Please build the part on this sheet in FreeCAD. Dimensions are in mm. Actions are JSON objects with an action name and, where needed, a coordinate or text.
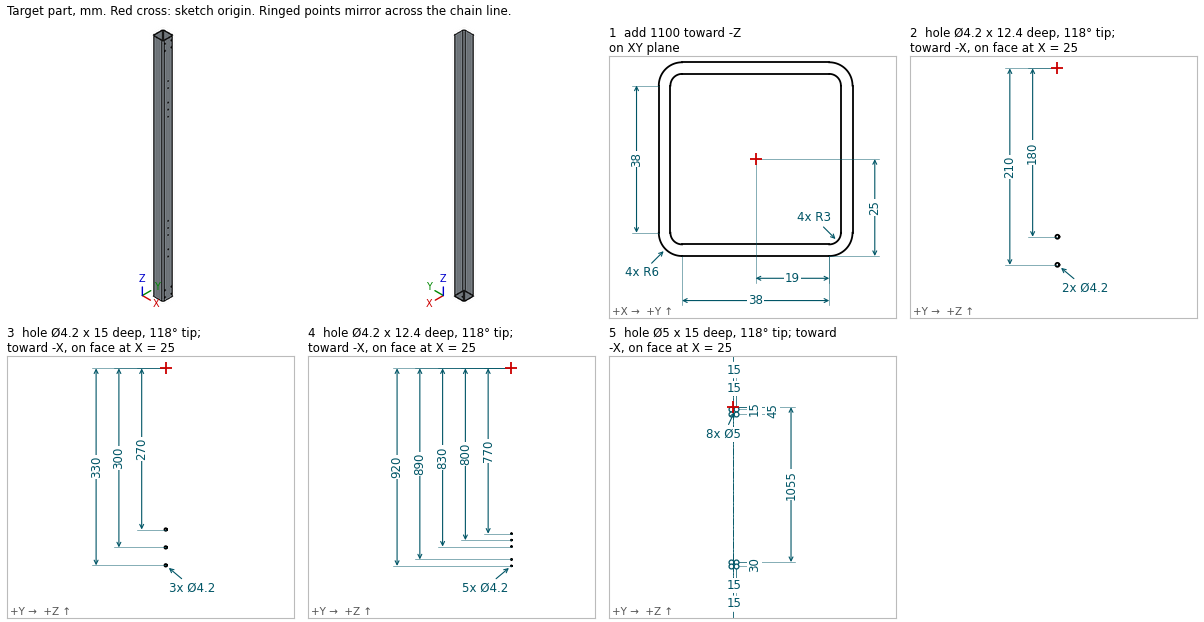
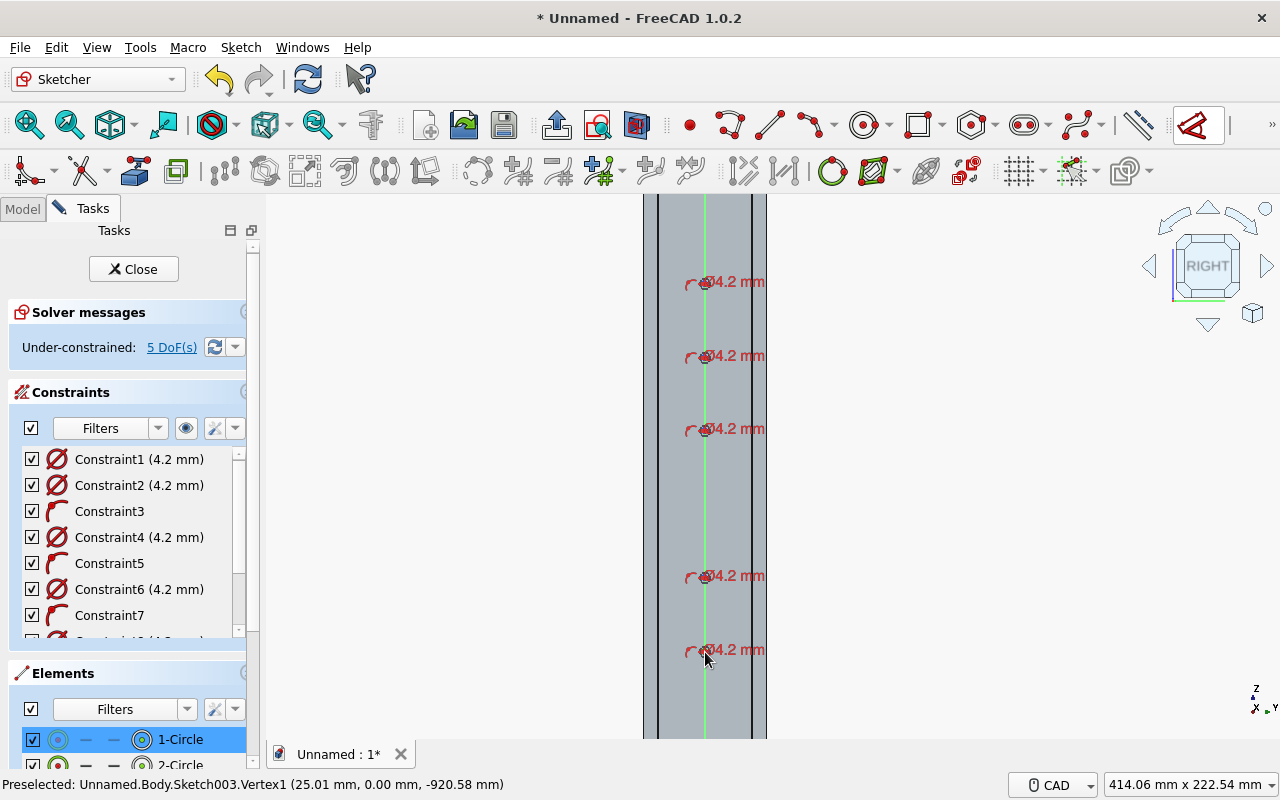
{"action": "key", "text": "i"}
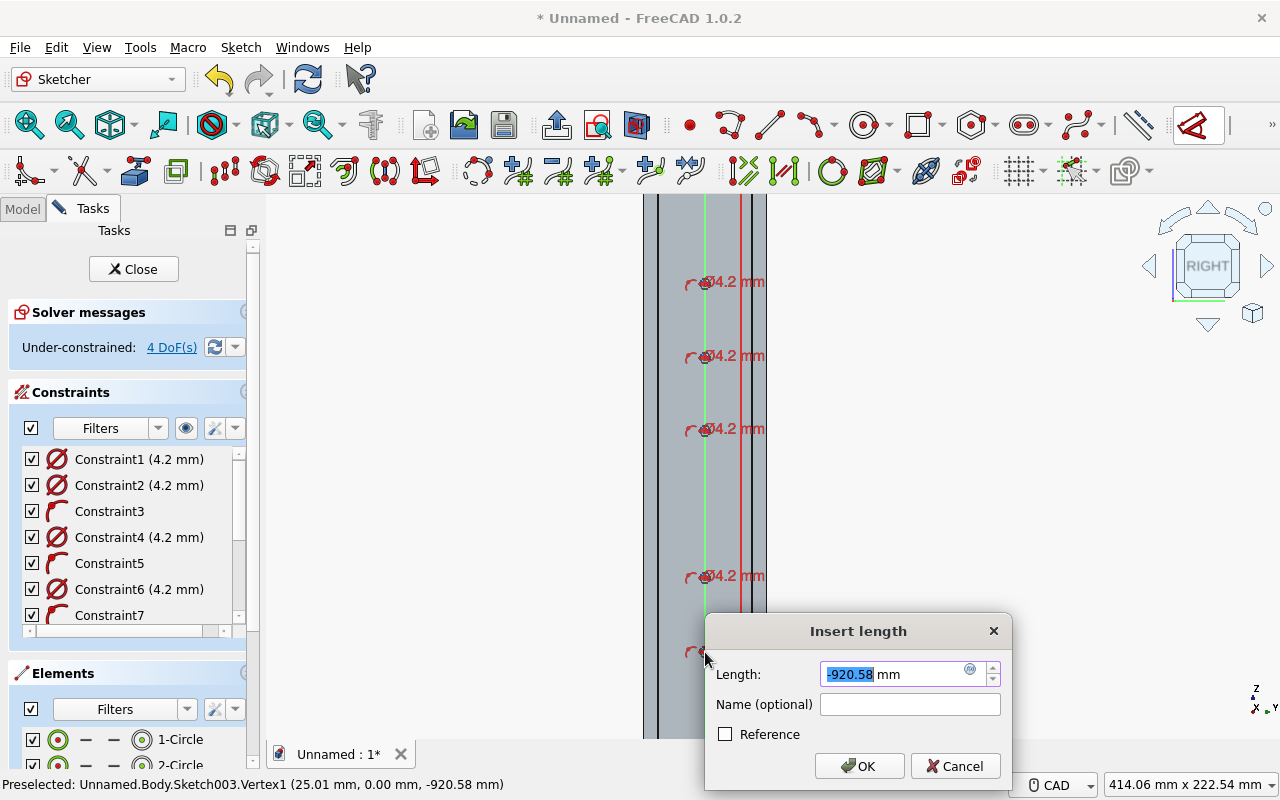
{"action": "type", "text": "-920"}
{"action": "key", "text": "Return"}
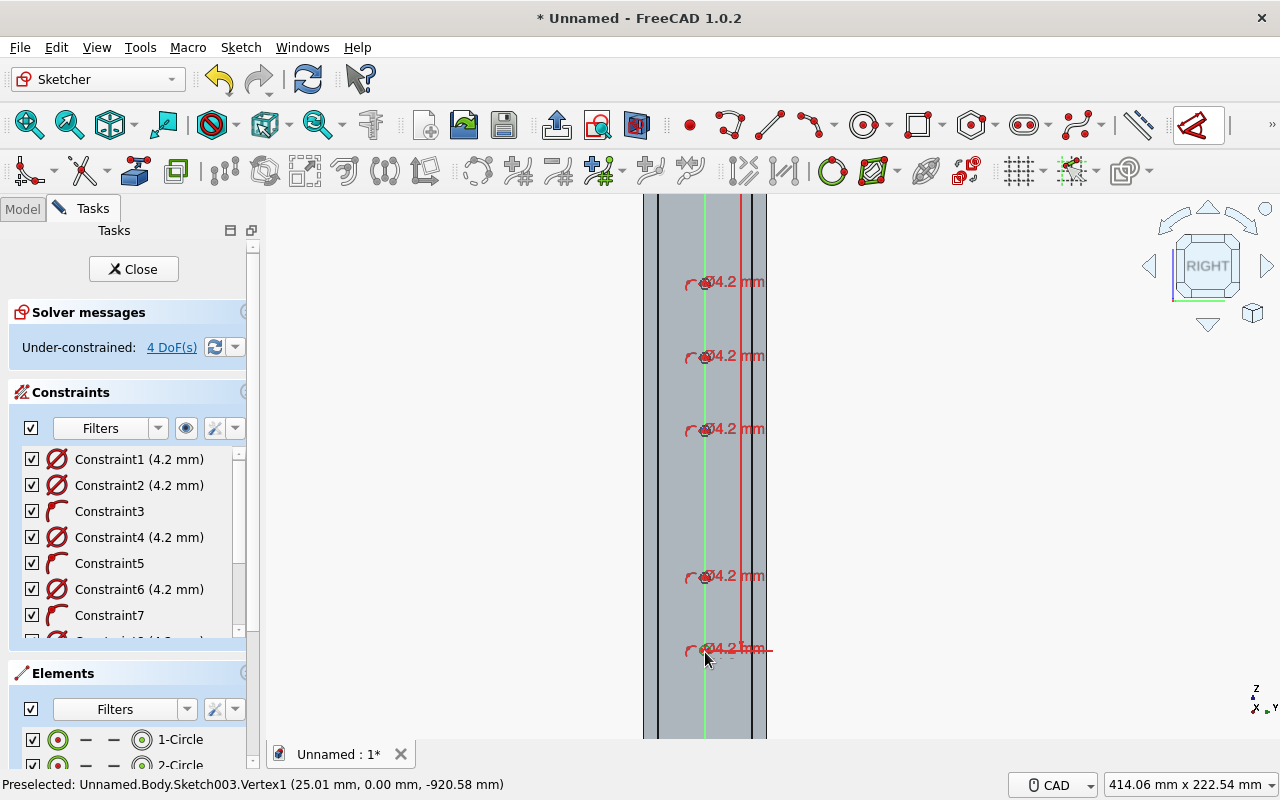
{"action": "left_click", "coordinate": [705, 578]}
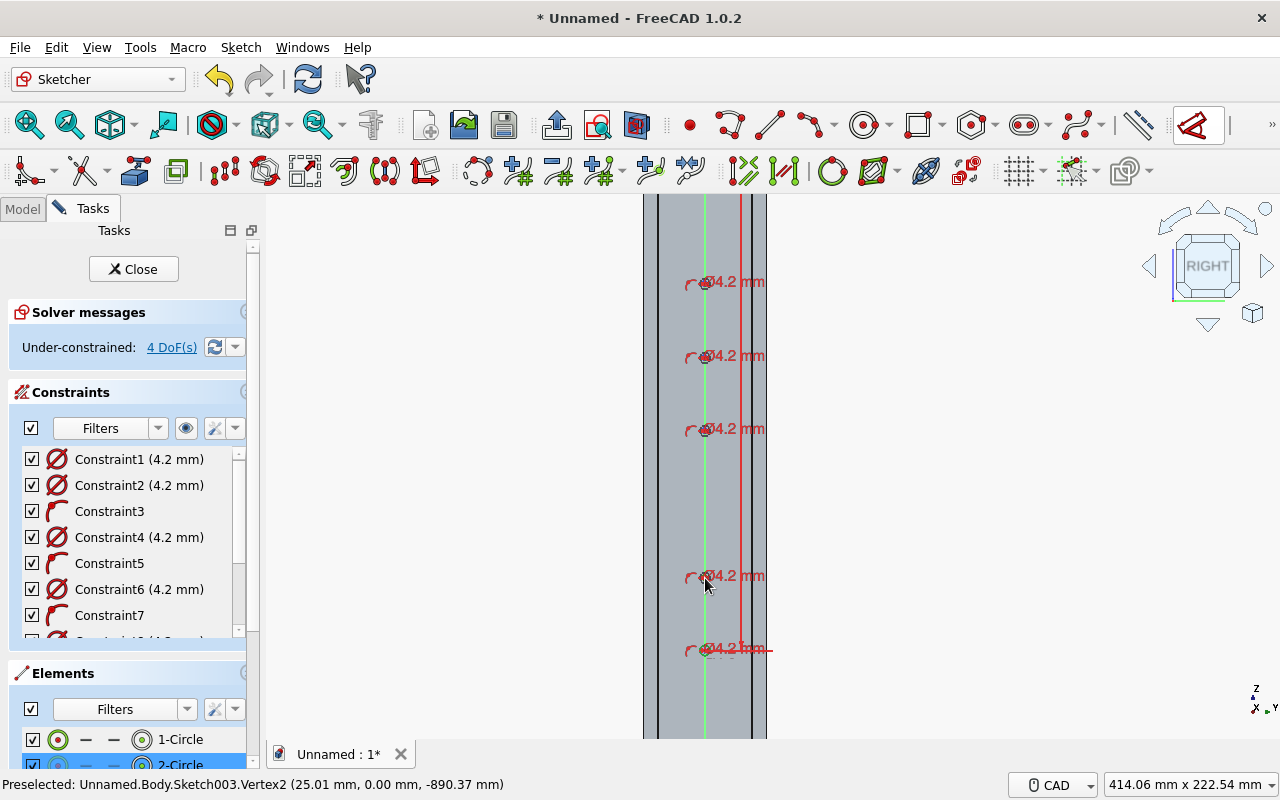
{"action": "key", "text": "i"}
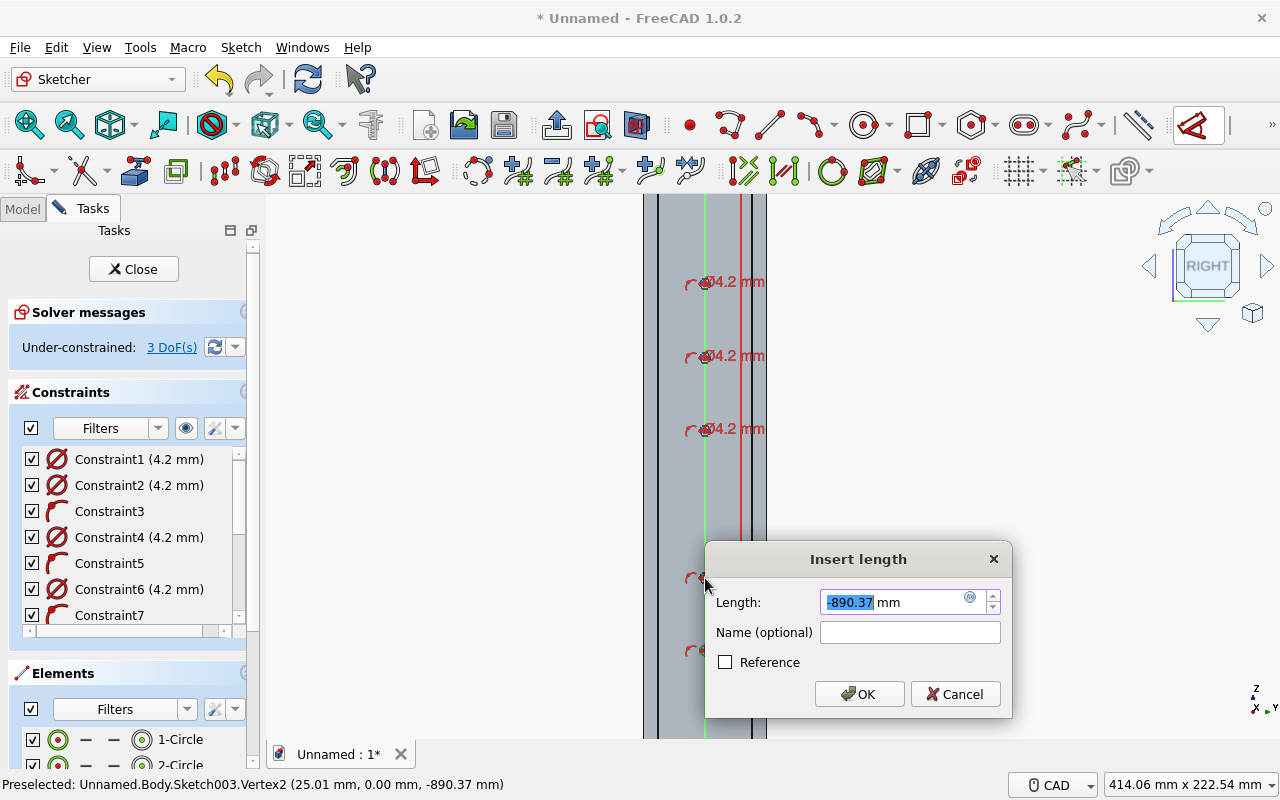
{"action": "type", "text": "-890"}
{"action": "key", "text": "Return"}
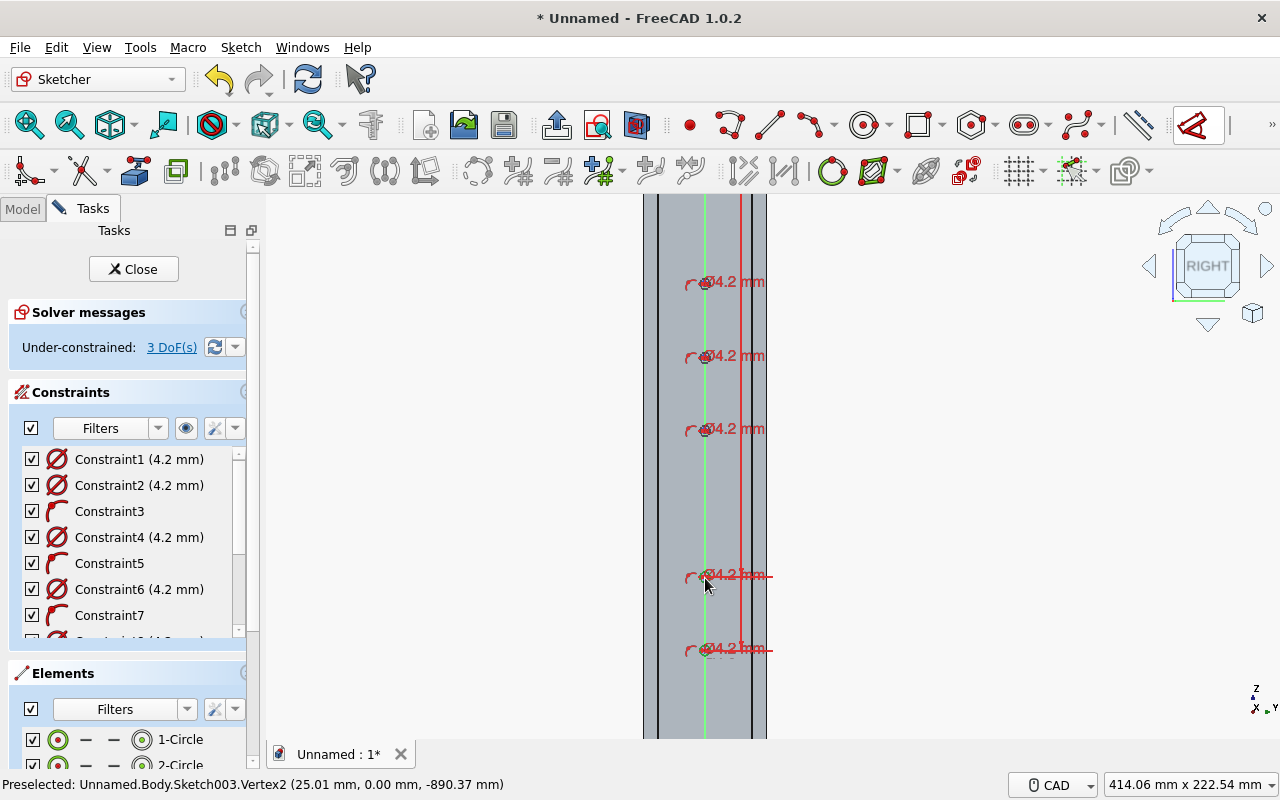
{"action": "left_click", "coordinate": [705, 431]}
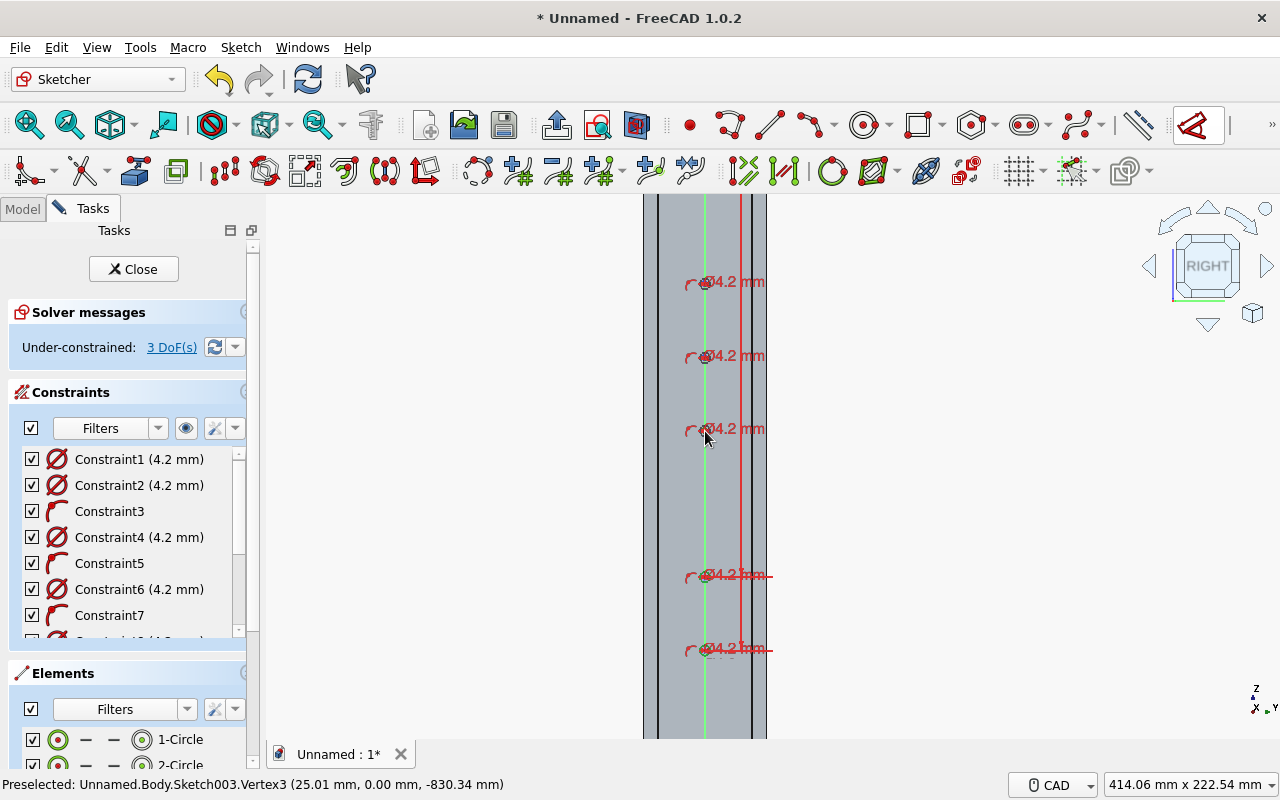
{"action": "left_click", "coordinate": [1218, 126]}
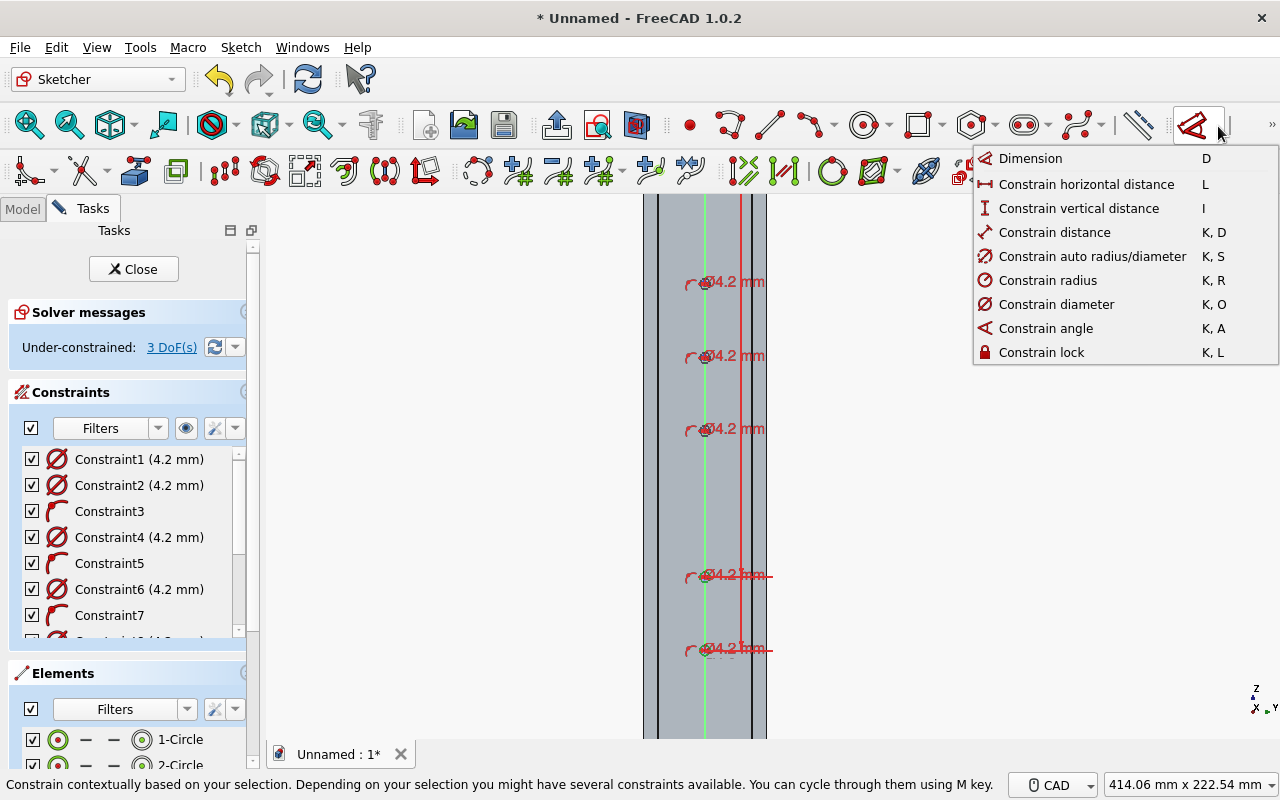
{"action": "left_click", "coordinate": [1126, 208]}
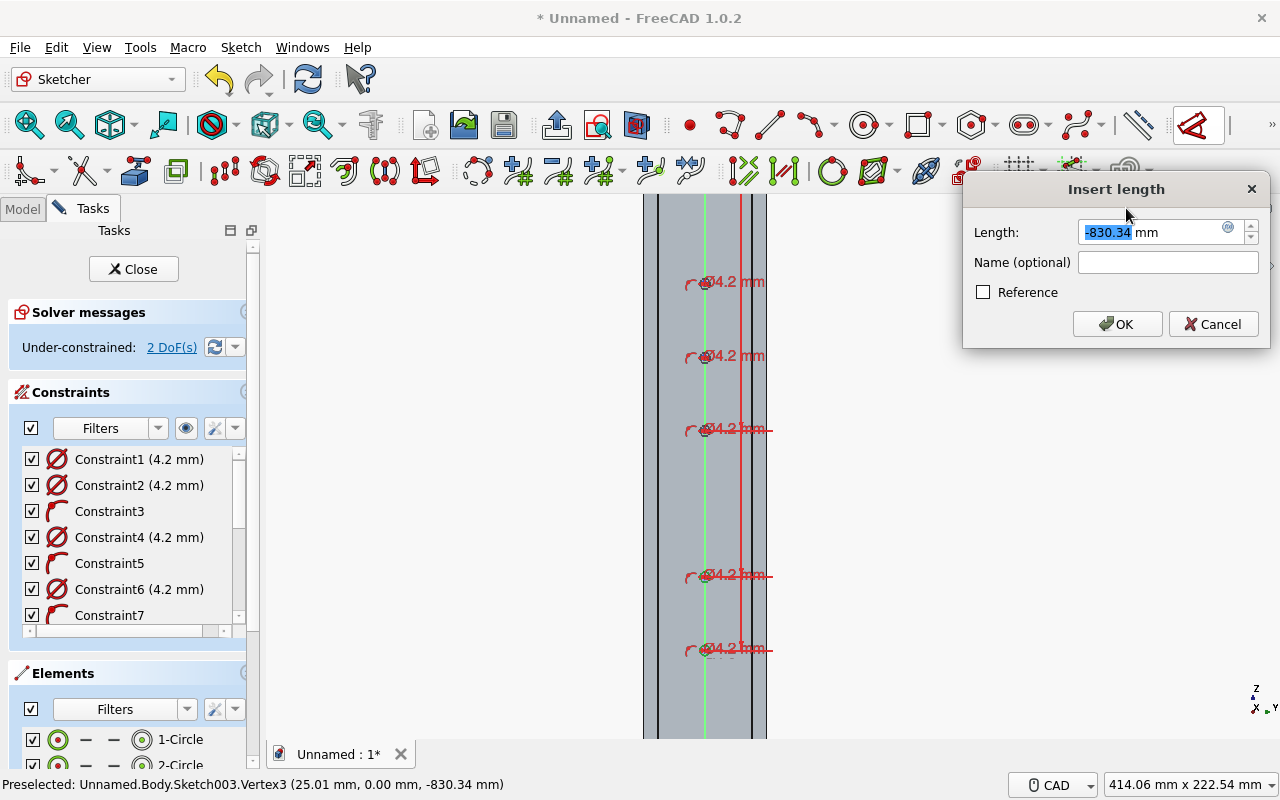
{"action": "type", "text": "-830"}
{"action": "key", "text": "Return"}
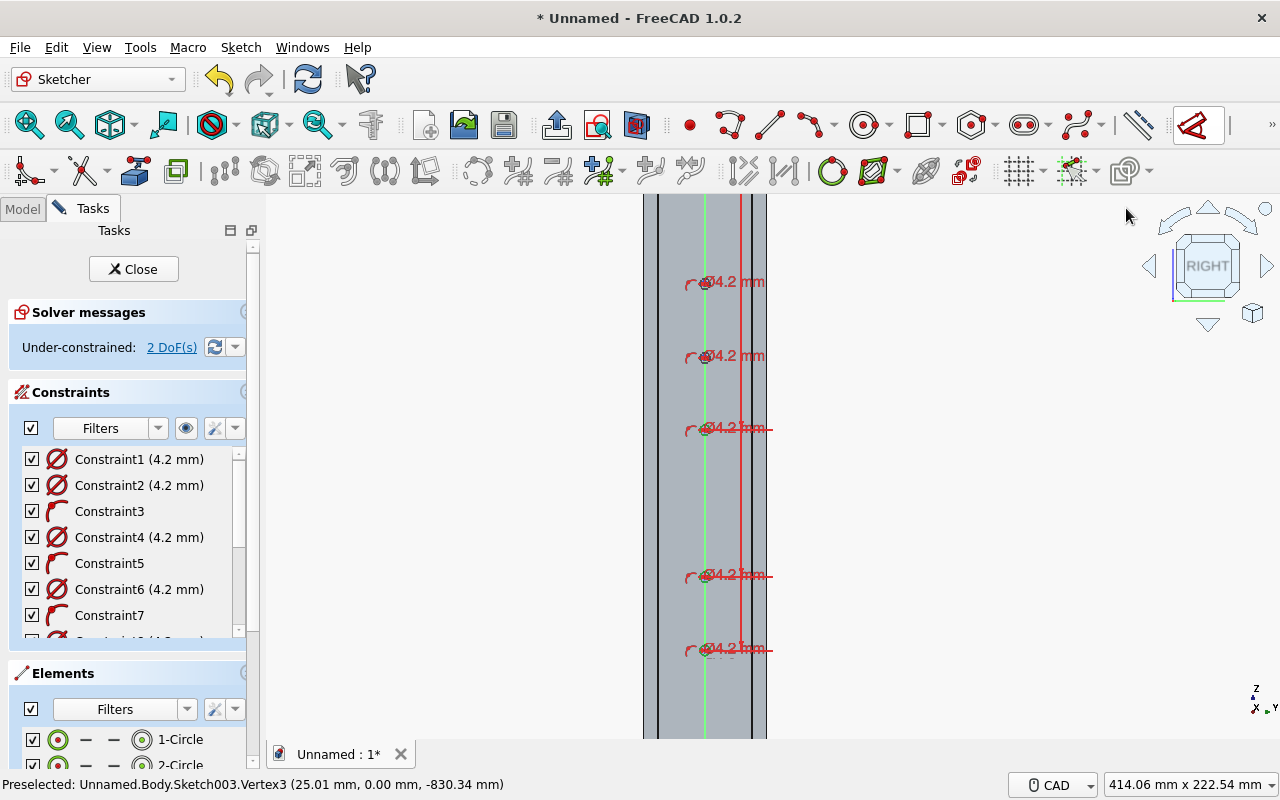
{"action": "left_click", "coordinate": [705, 358]}